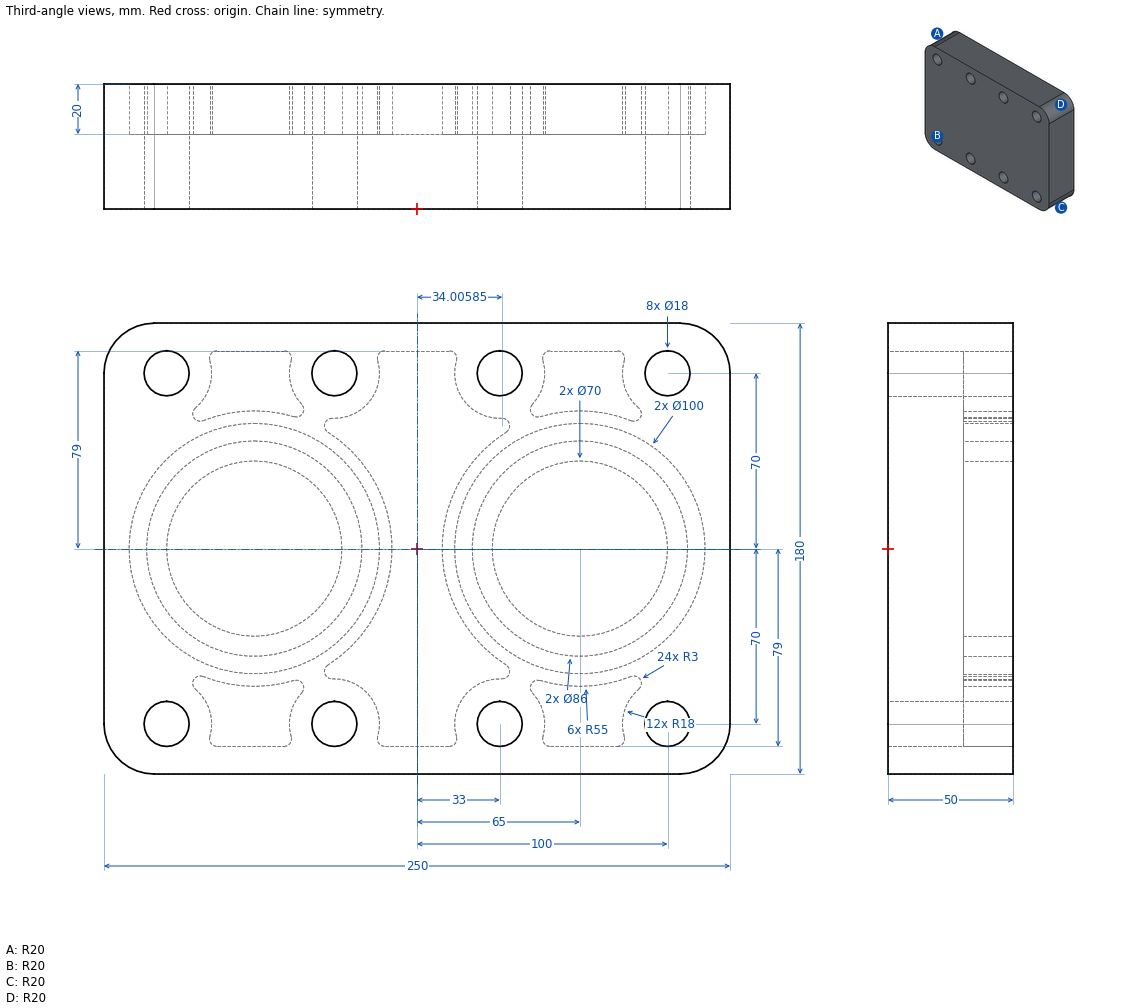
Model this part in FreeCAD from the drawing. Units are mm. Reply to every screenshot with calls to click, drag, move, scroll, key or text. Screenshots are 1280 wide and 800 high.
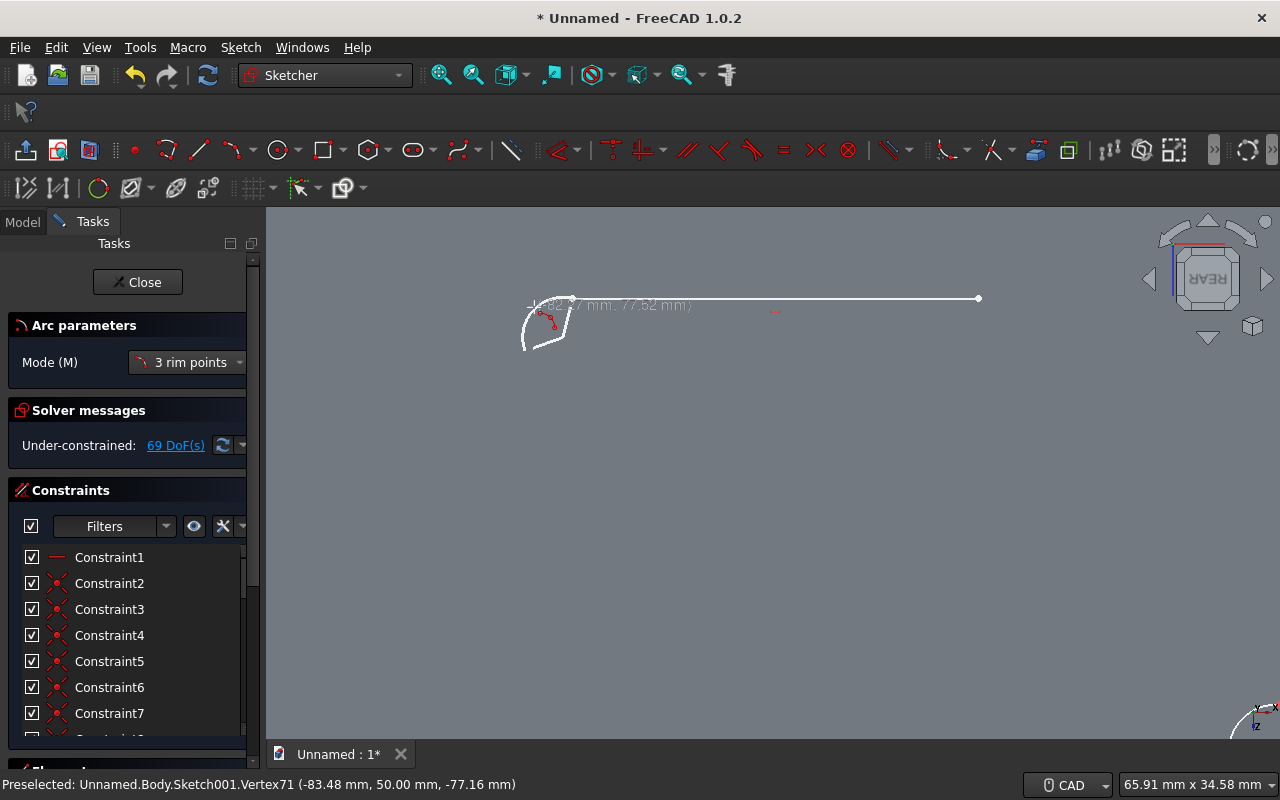
click(533, 306)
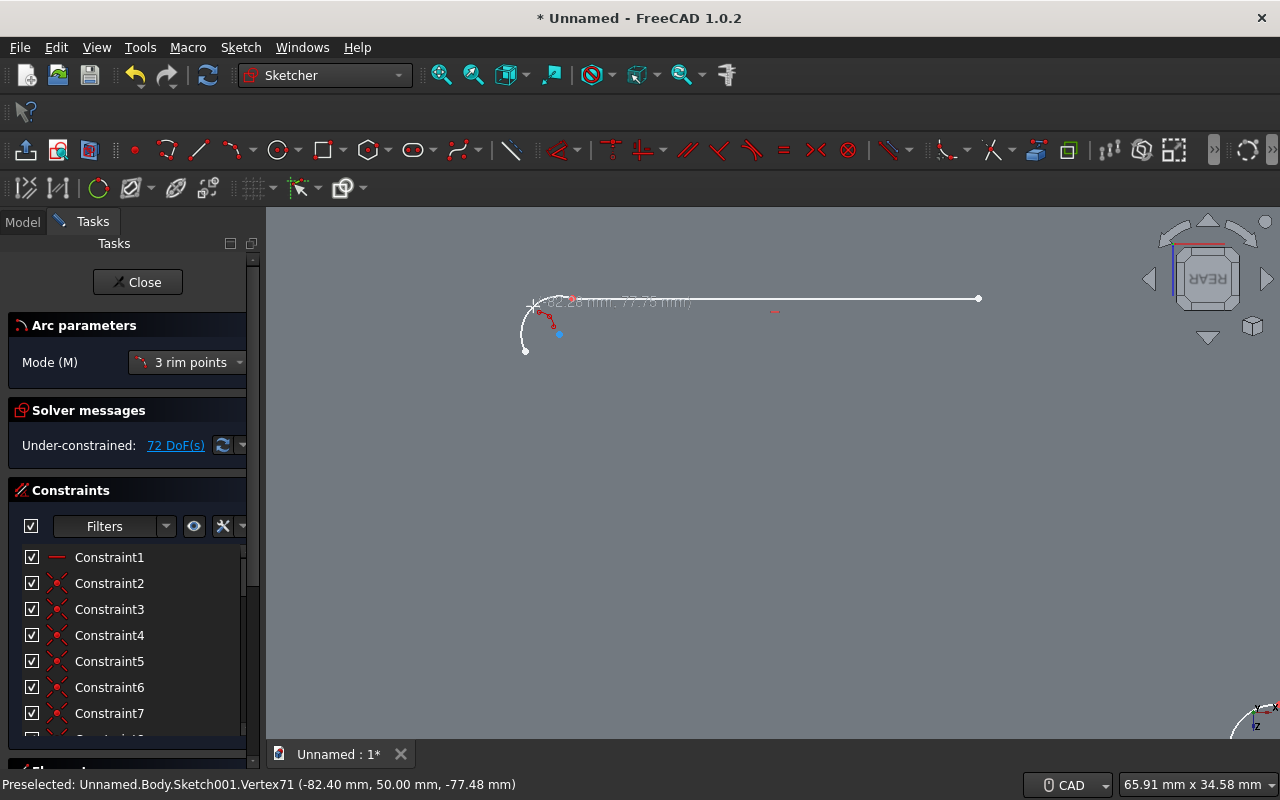
scroll(533, 312, down, 10)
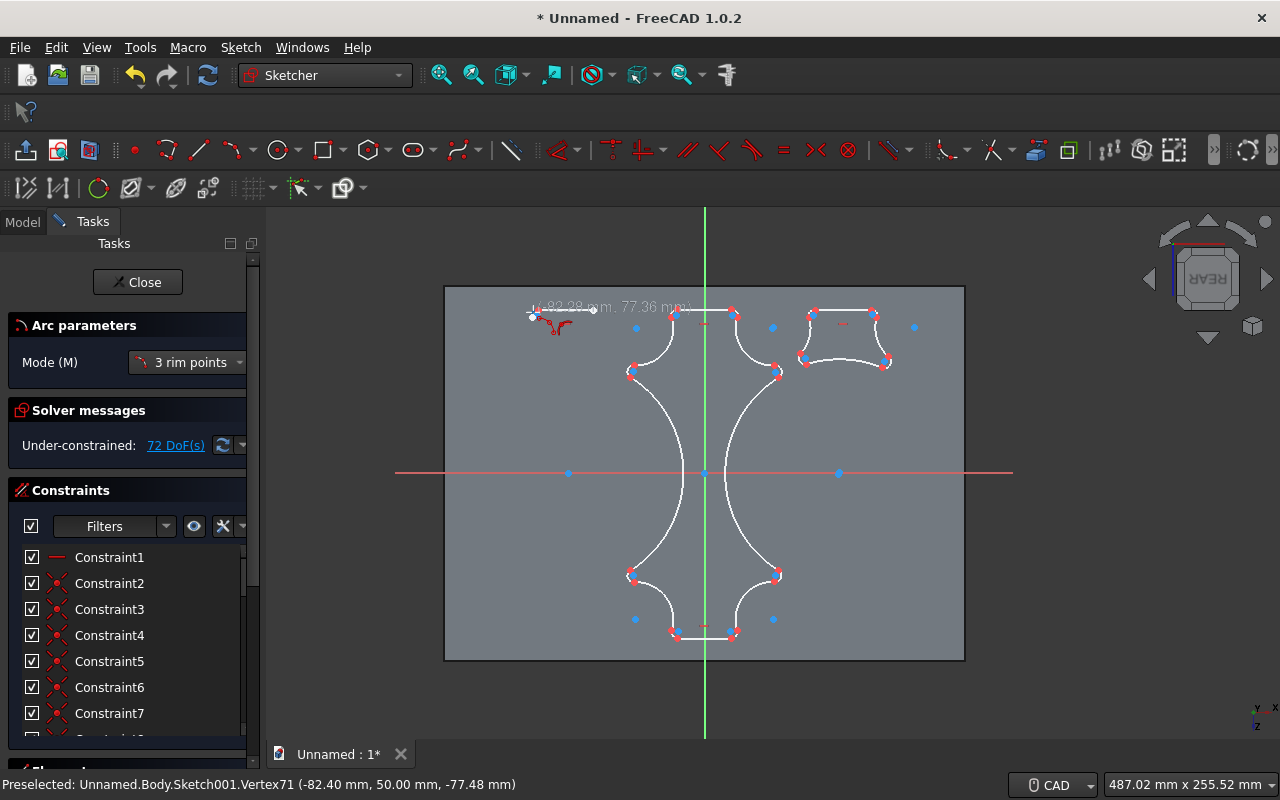
scroll(532, 317, up, 5)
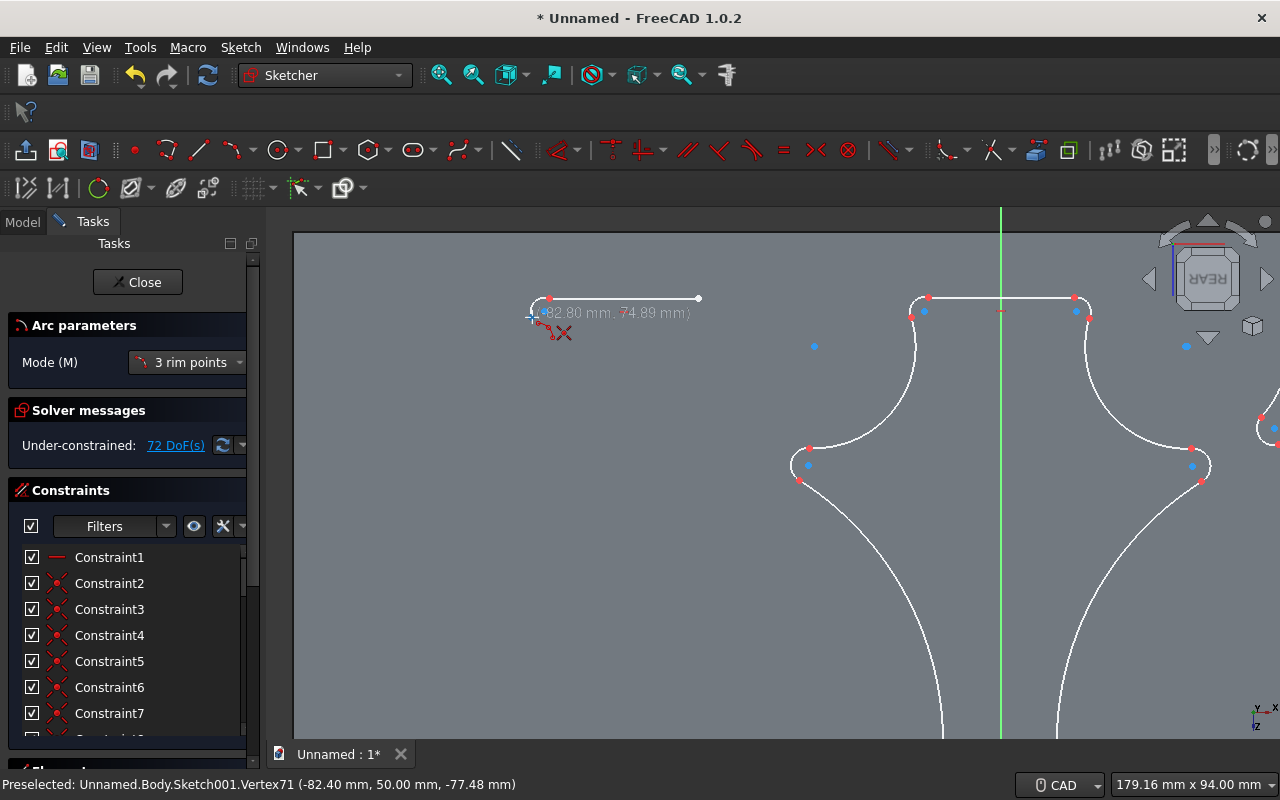
click(532, 318)
click(500, 424)
click(532, 375)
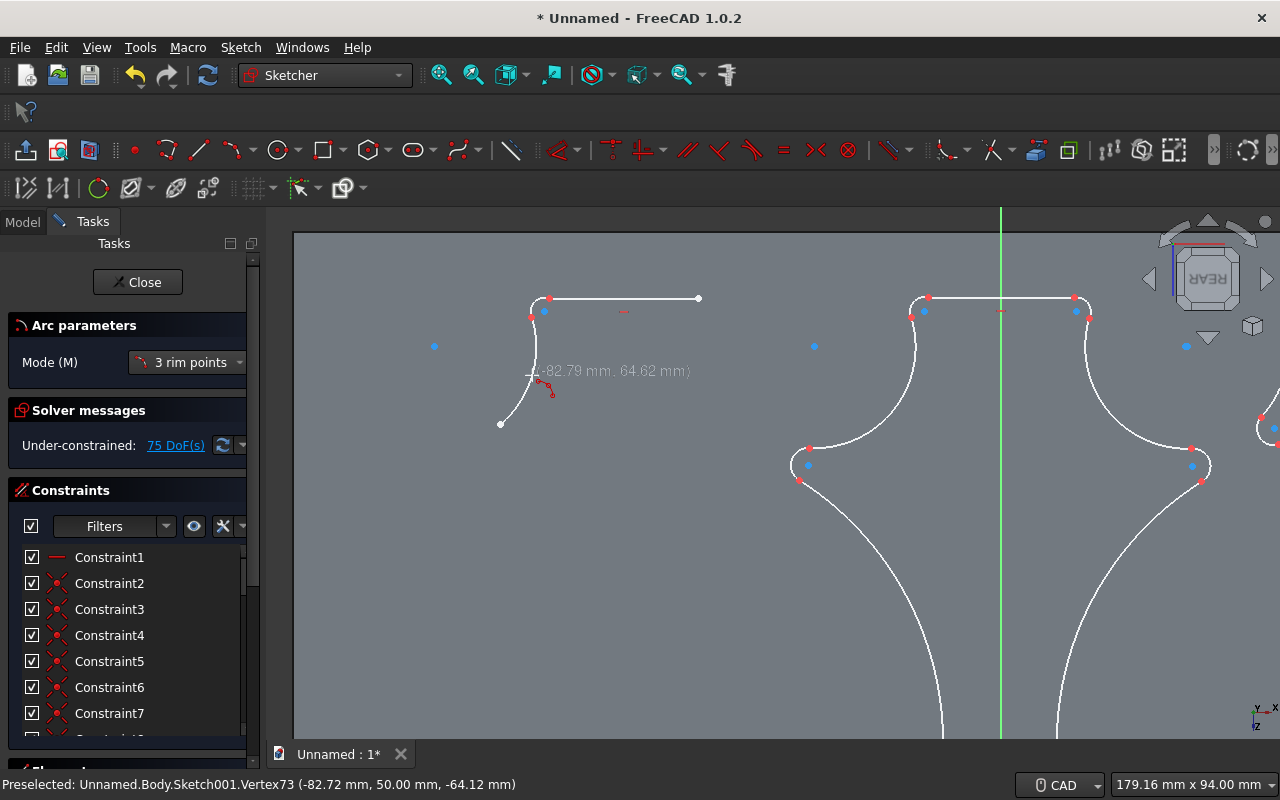
click(500, 425)
click(517, 453)
click(496, 446)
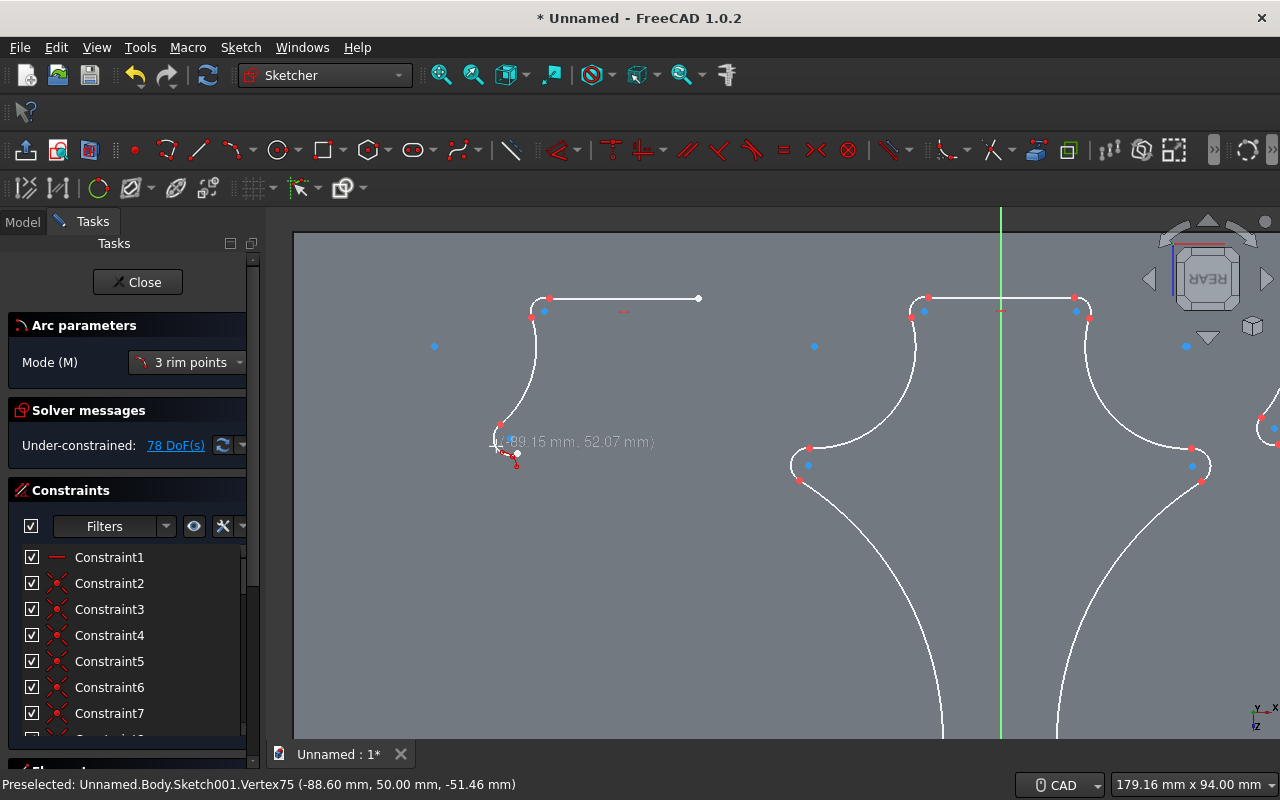
click(517, 454)
click(723, 444)
click(619, 431)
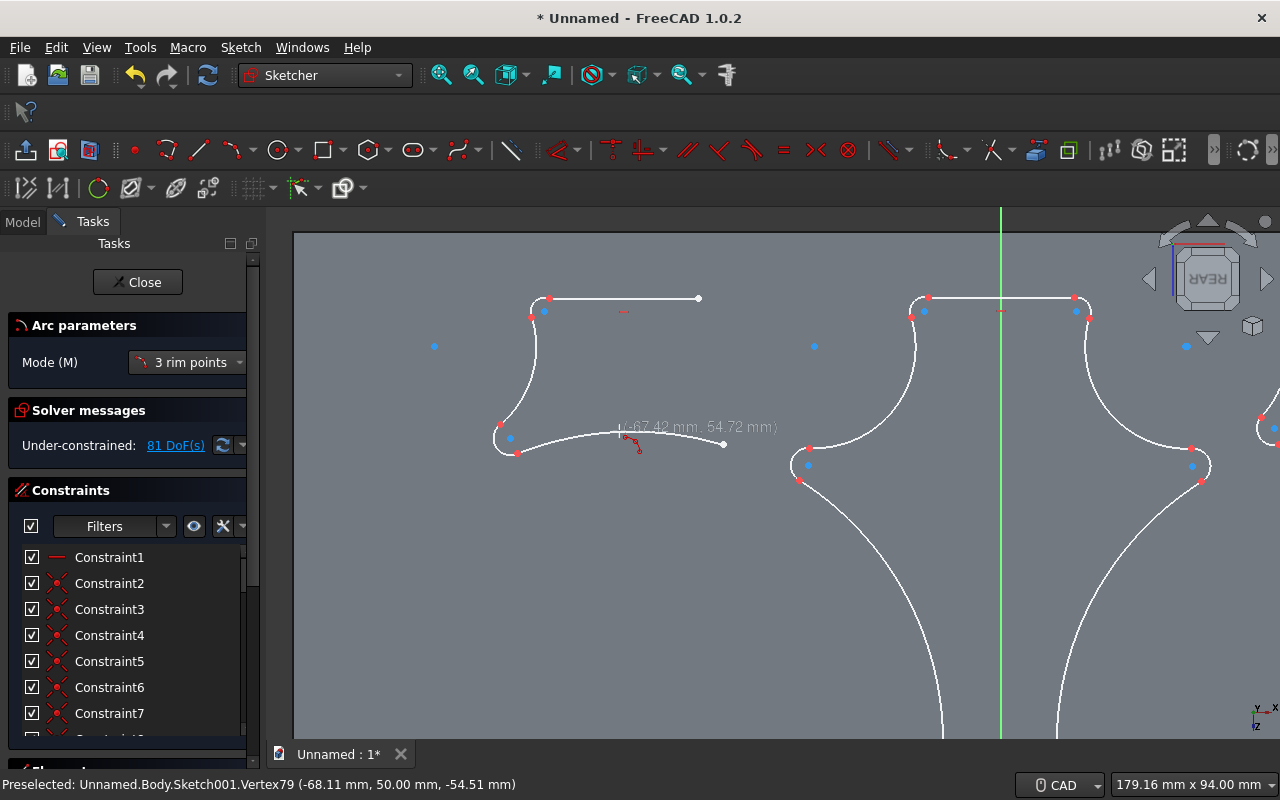
click(723, 445)
click(740, 416)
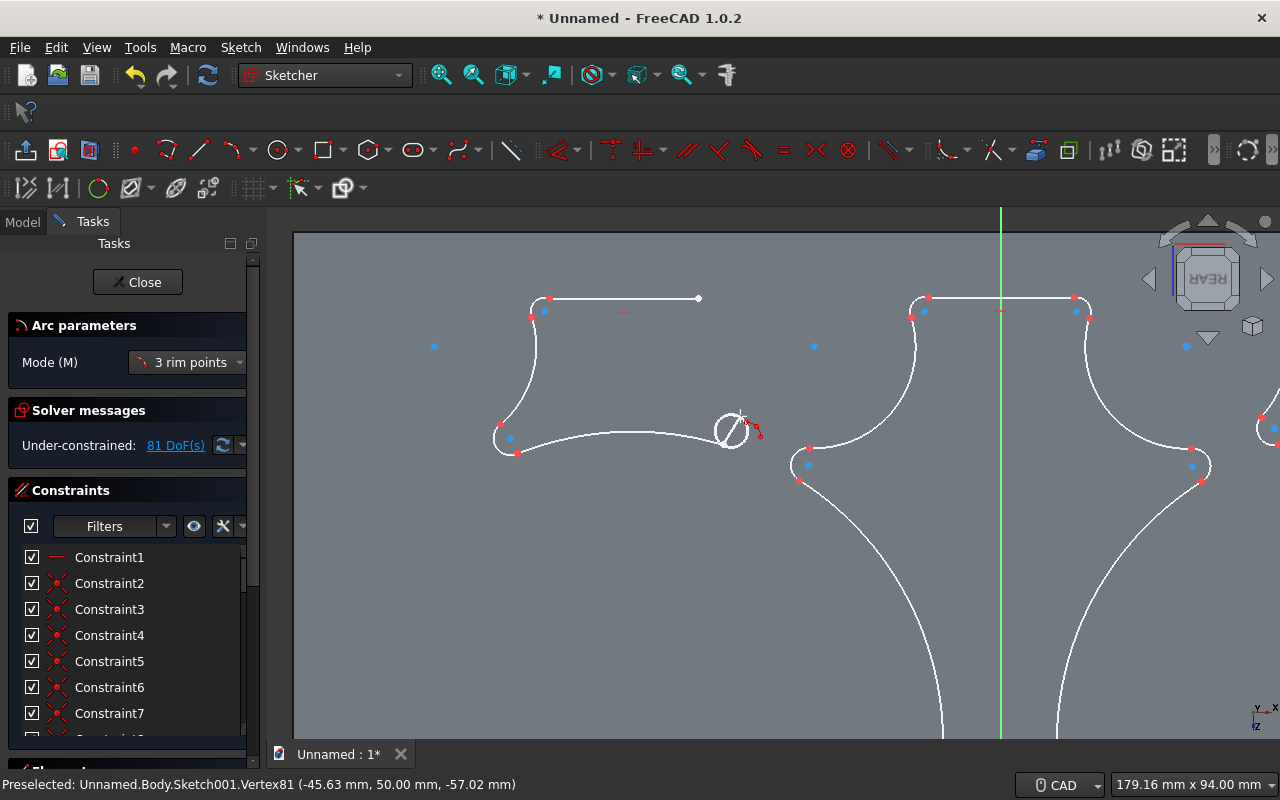
scroll(742, 436, up, 2)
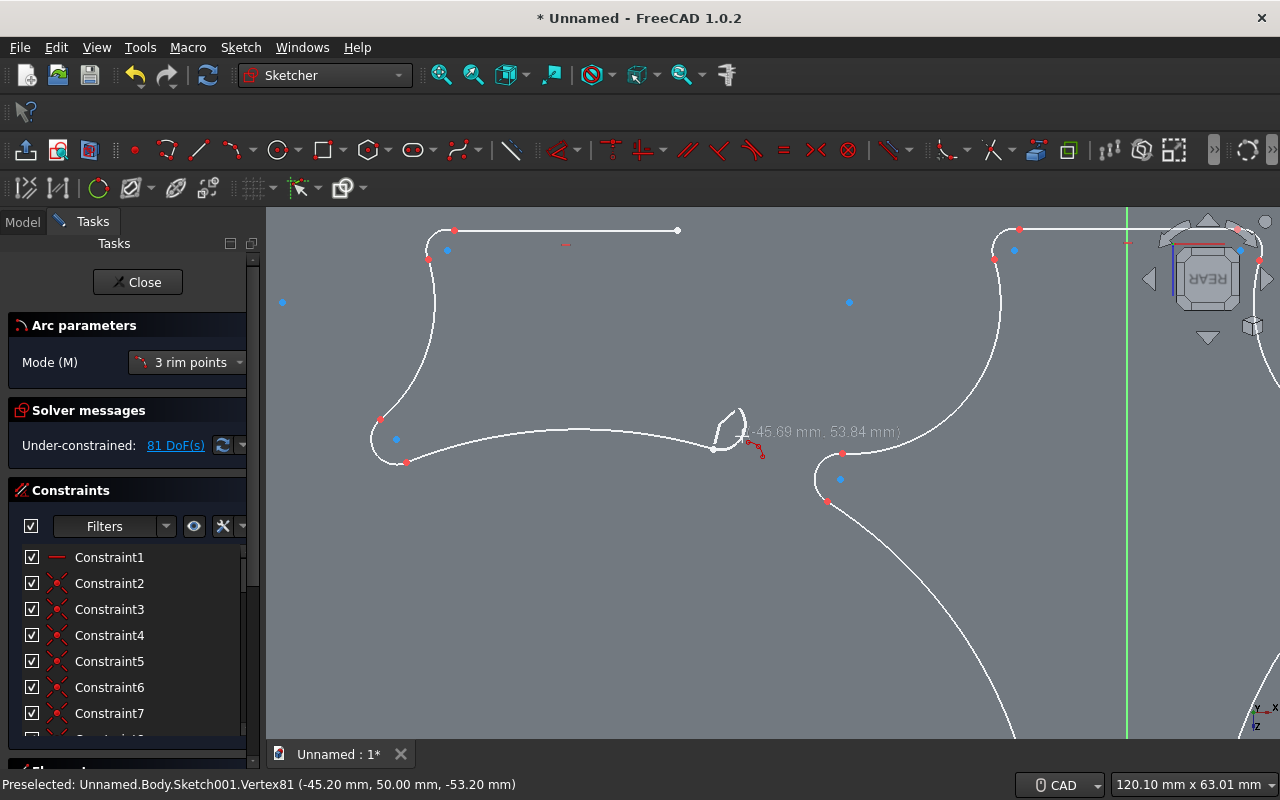
click(742, 436)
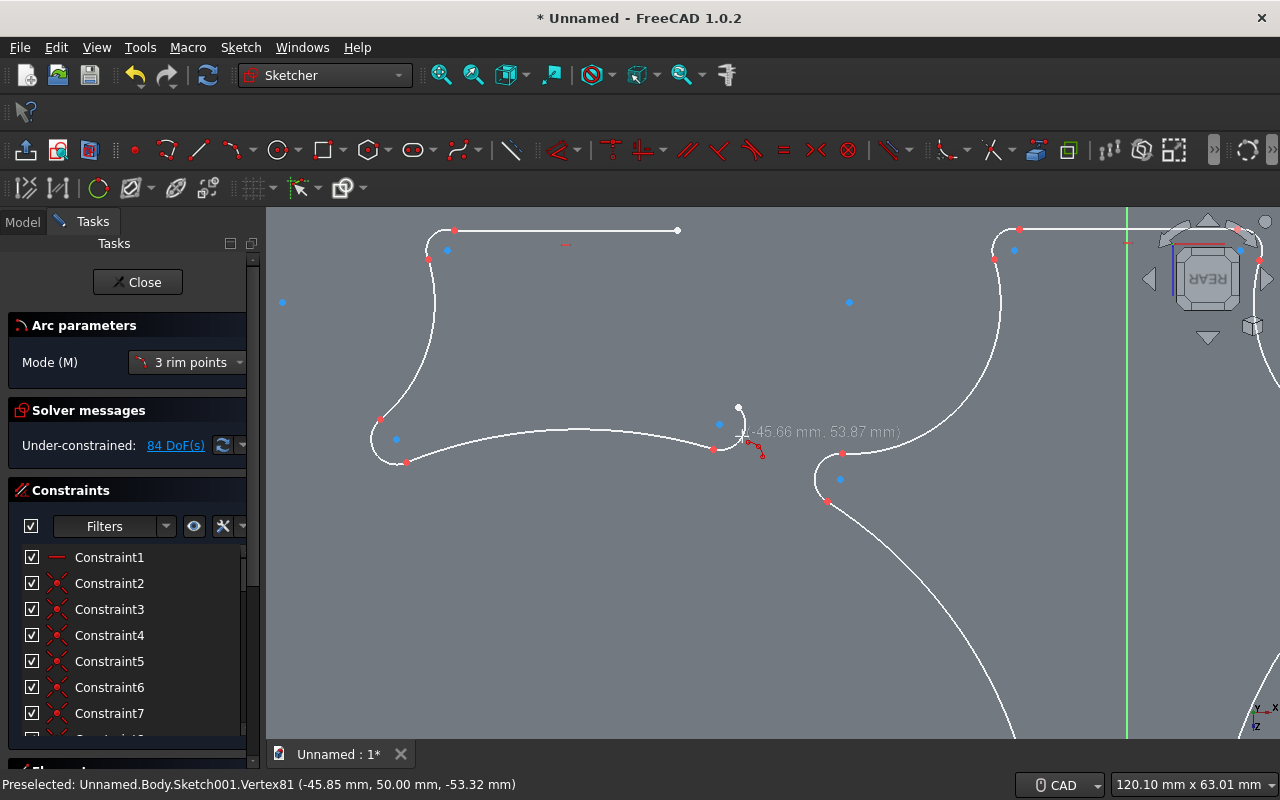
click(739, 407)
click(703, 257)
click(701, 336)